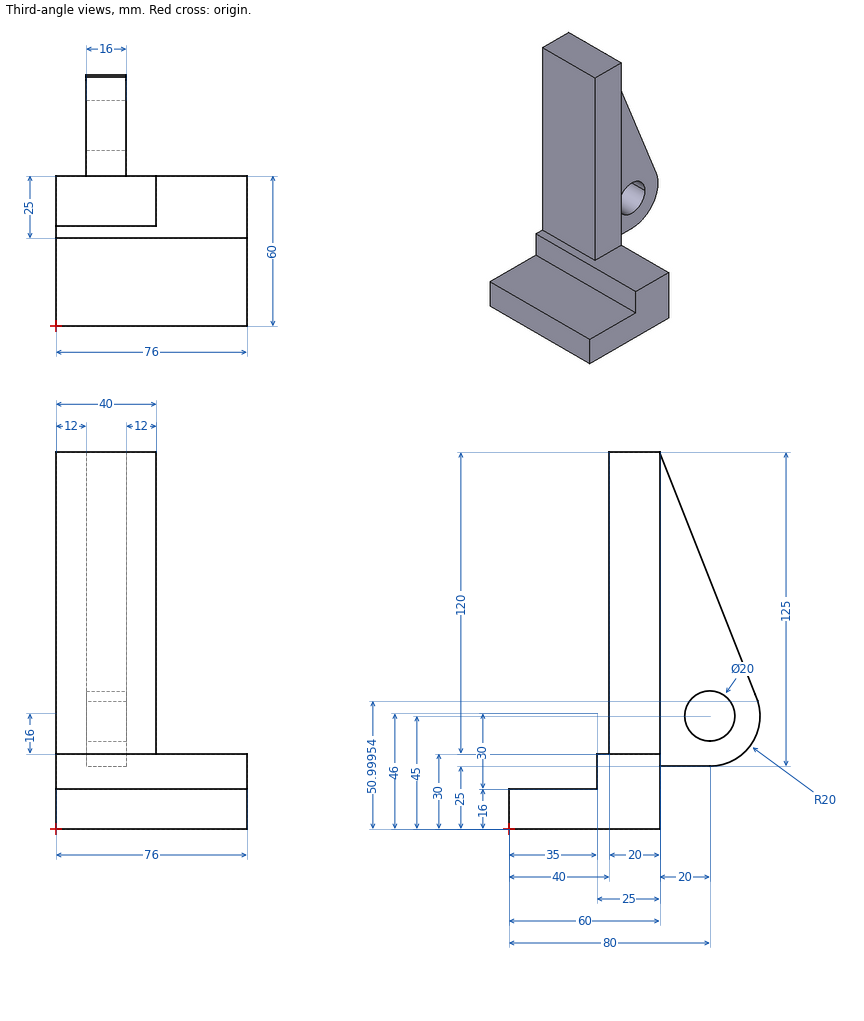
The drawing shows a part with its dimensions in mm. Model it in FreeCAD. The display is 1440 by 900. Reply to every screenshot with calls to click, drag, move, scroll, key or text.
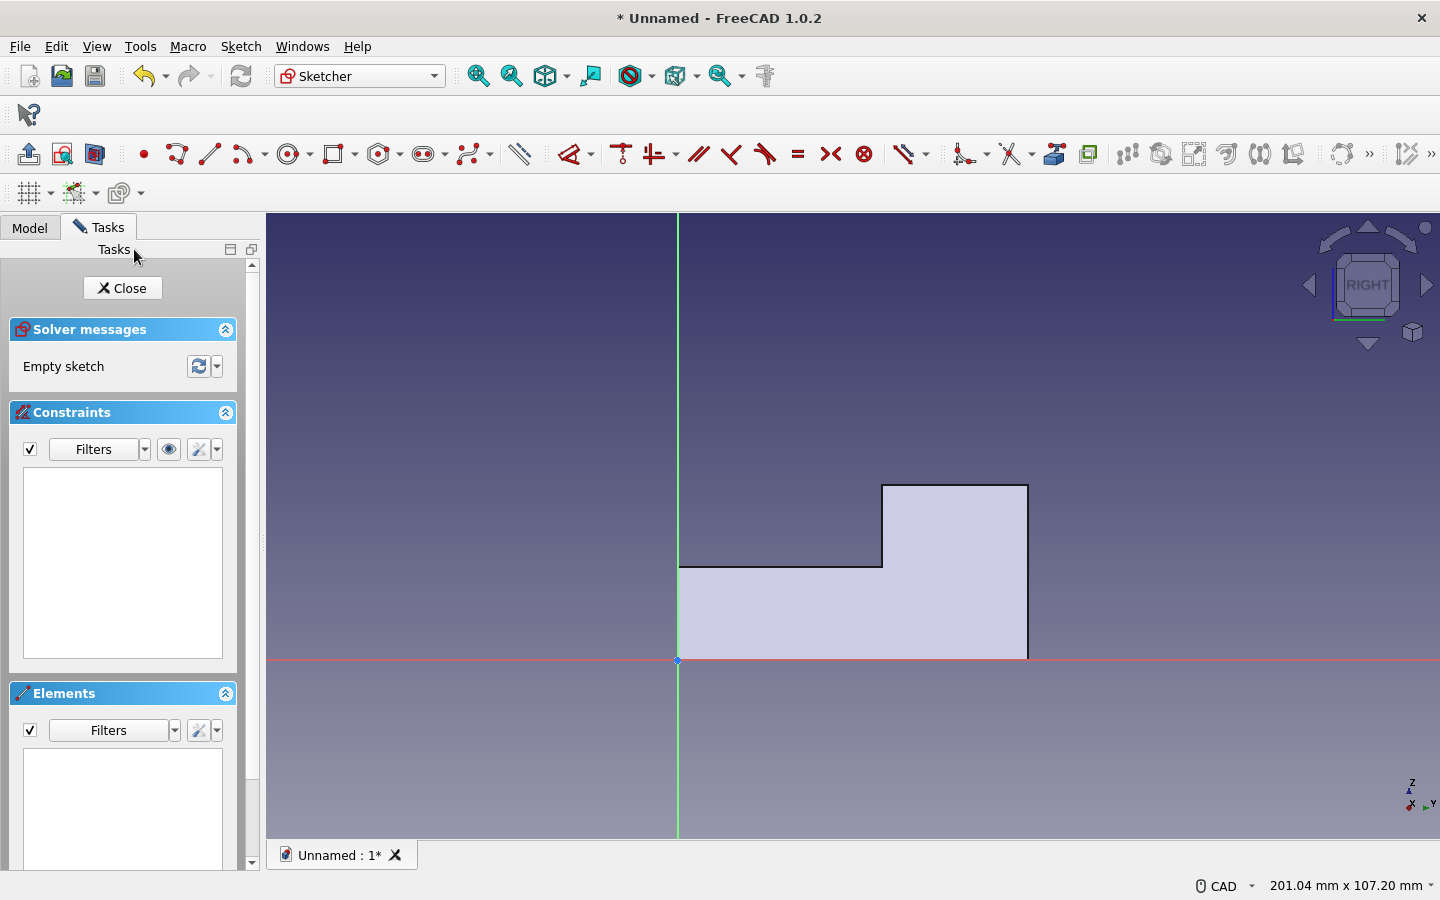
scroll(729, 774, down, 4)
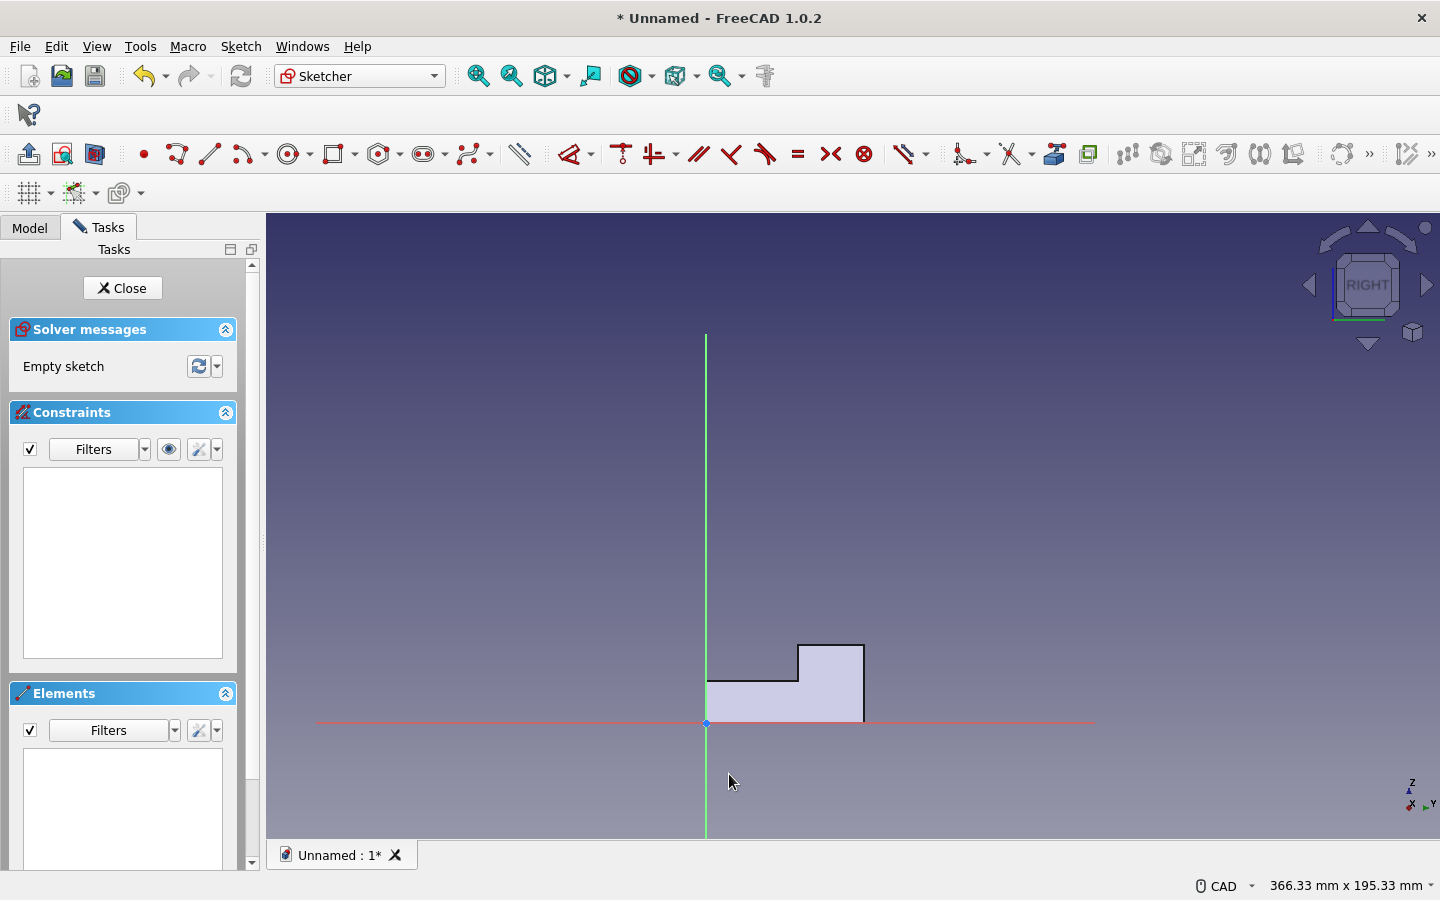
key(g)
key(r)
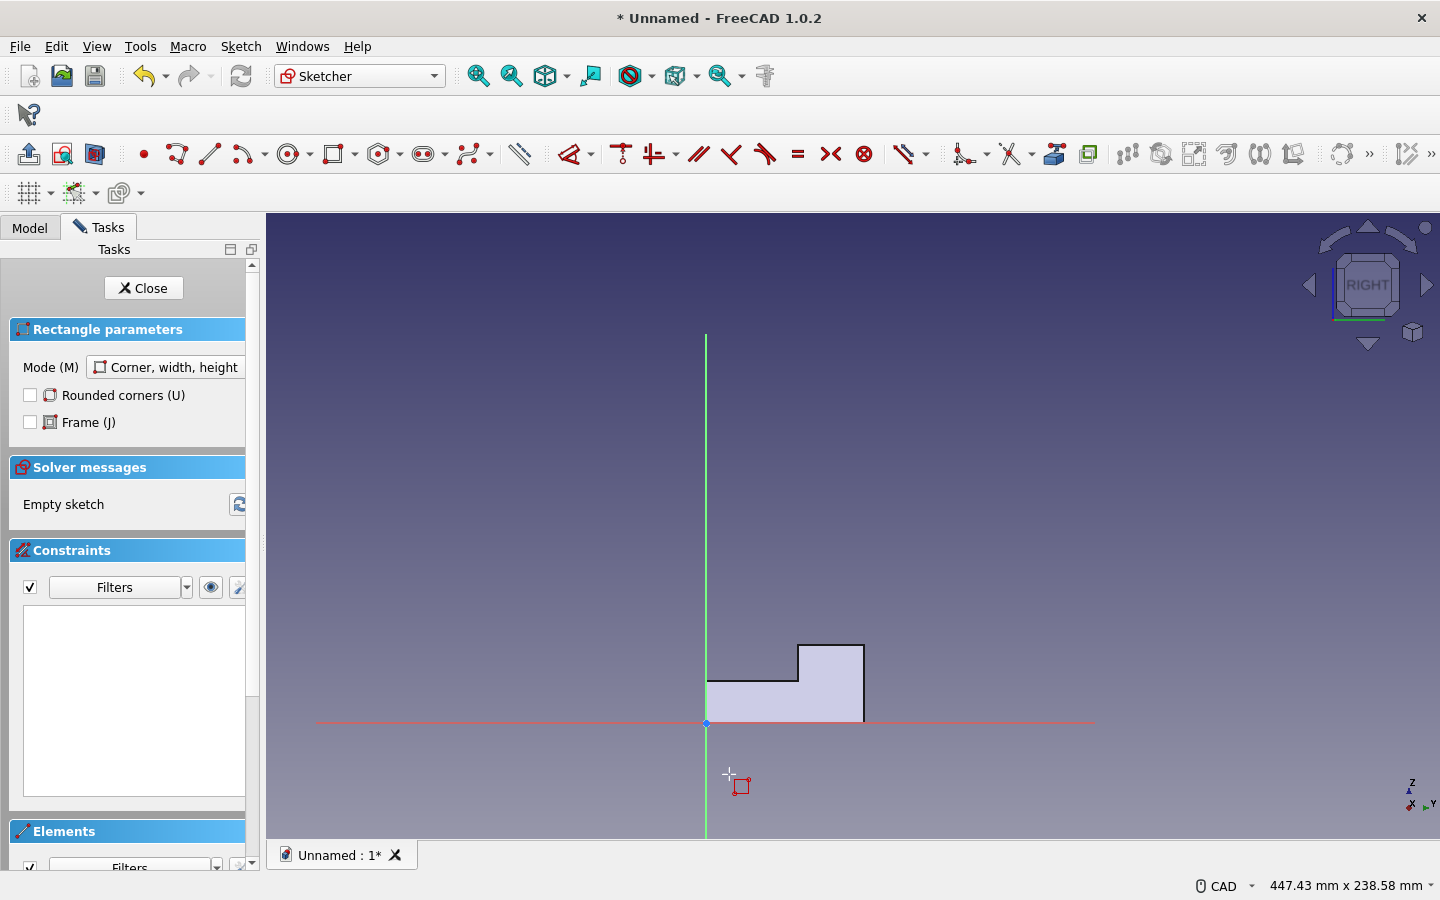
click(811, 330)
click(864, 645)
key(Escape)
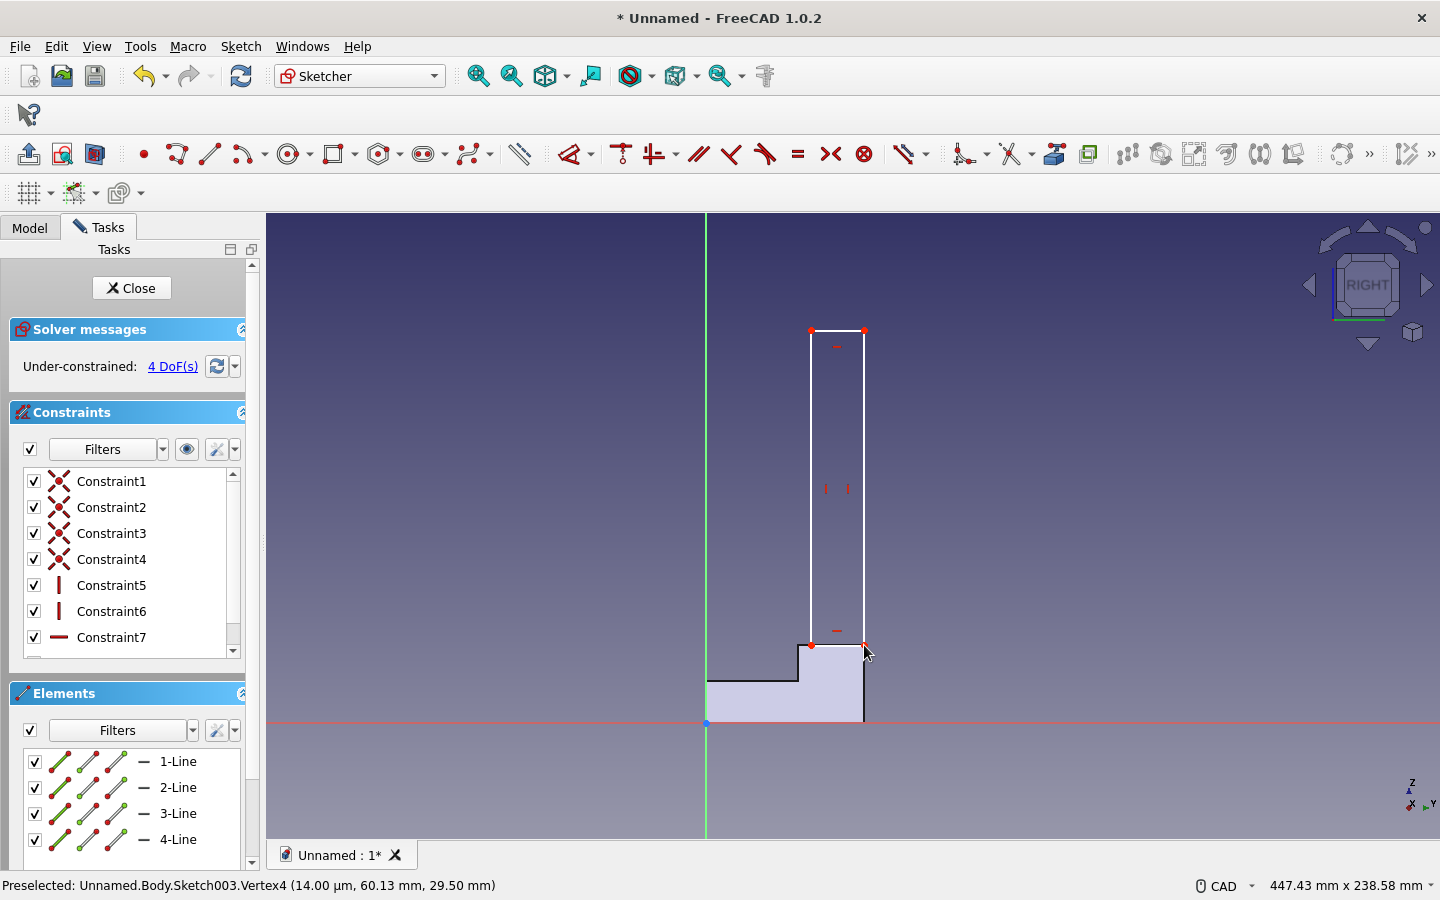
click(568, 154)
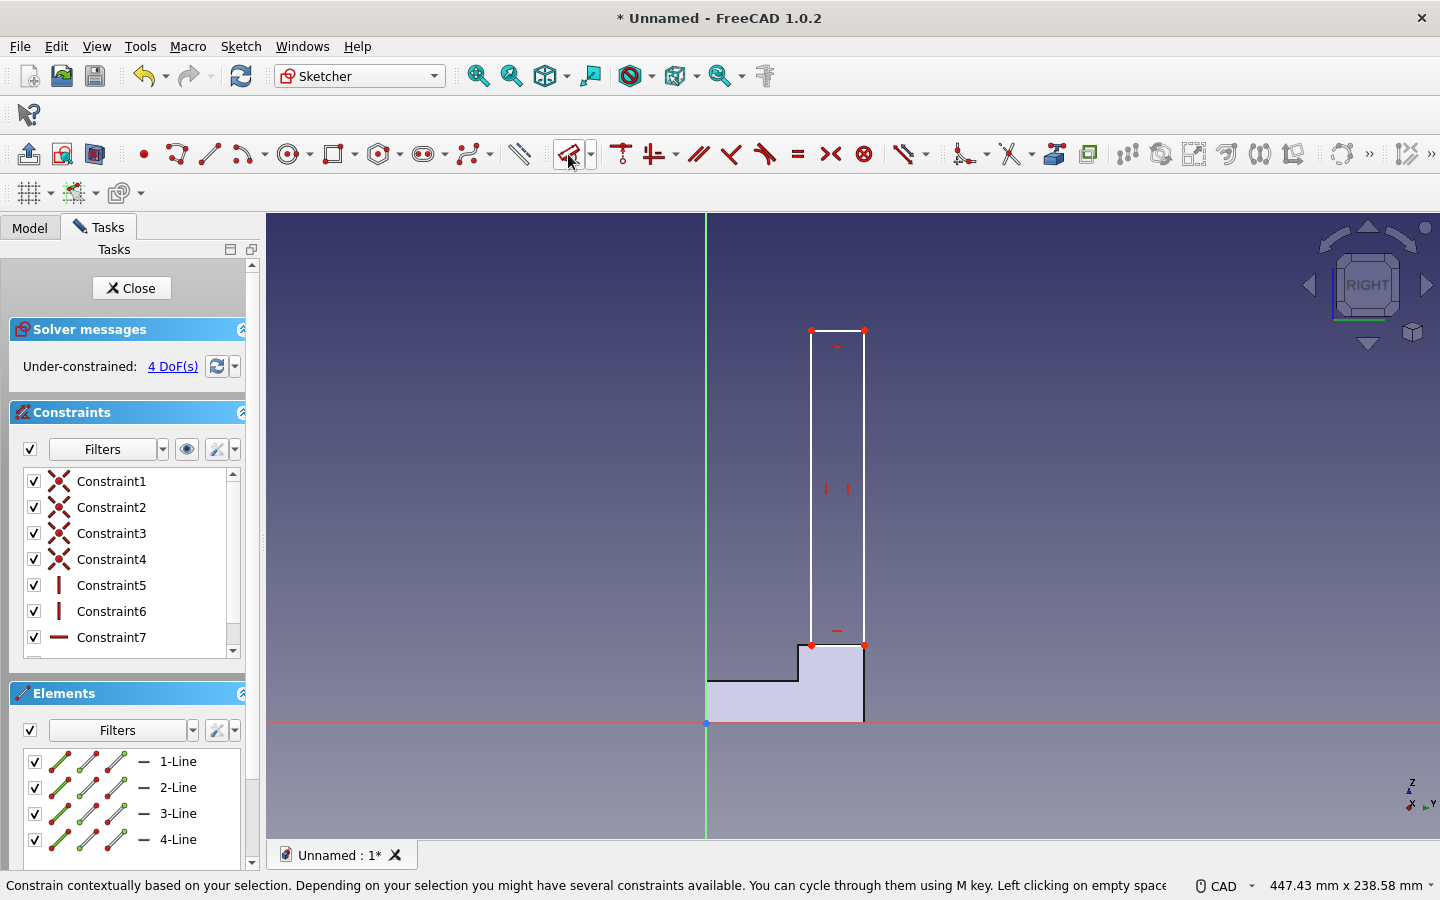
click(827, 646)
click(837, 680)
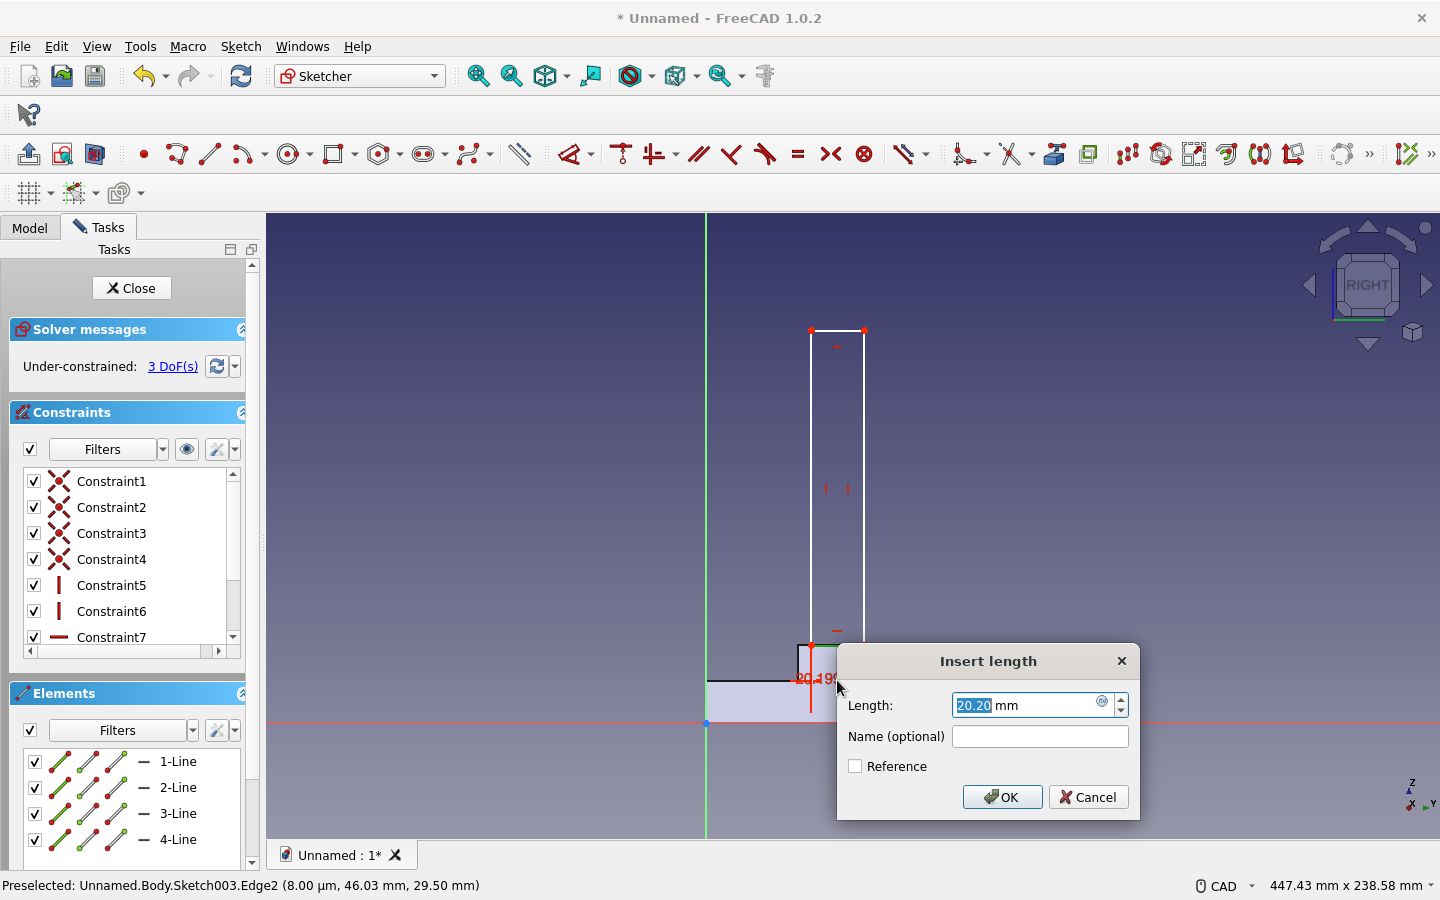
text(20)
key(Return)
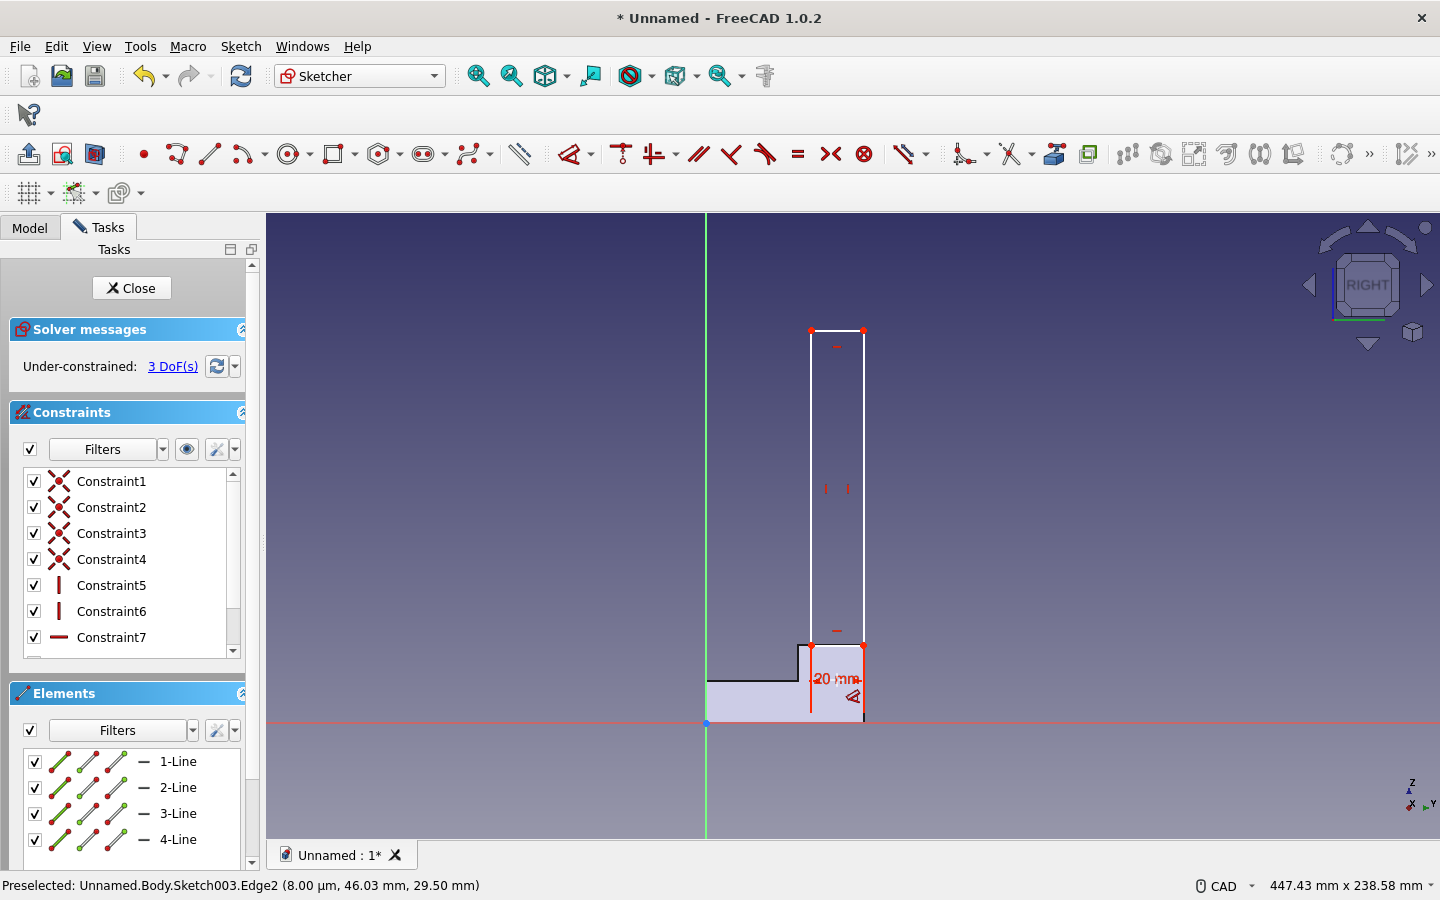
click(811, 425)
click(845, 488)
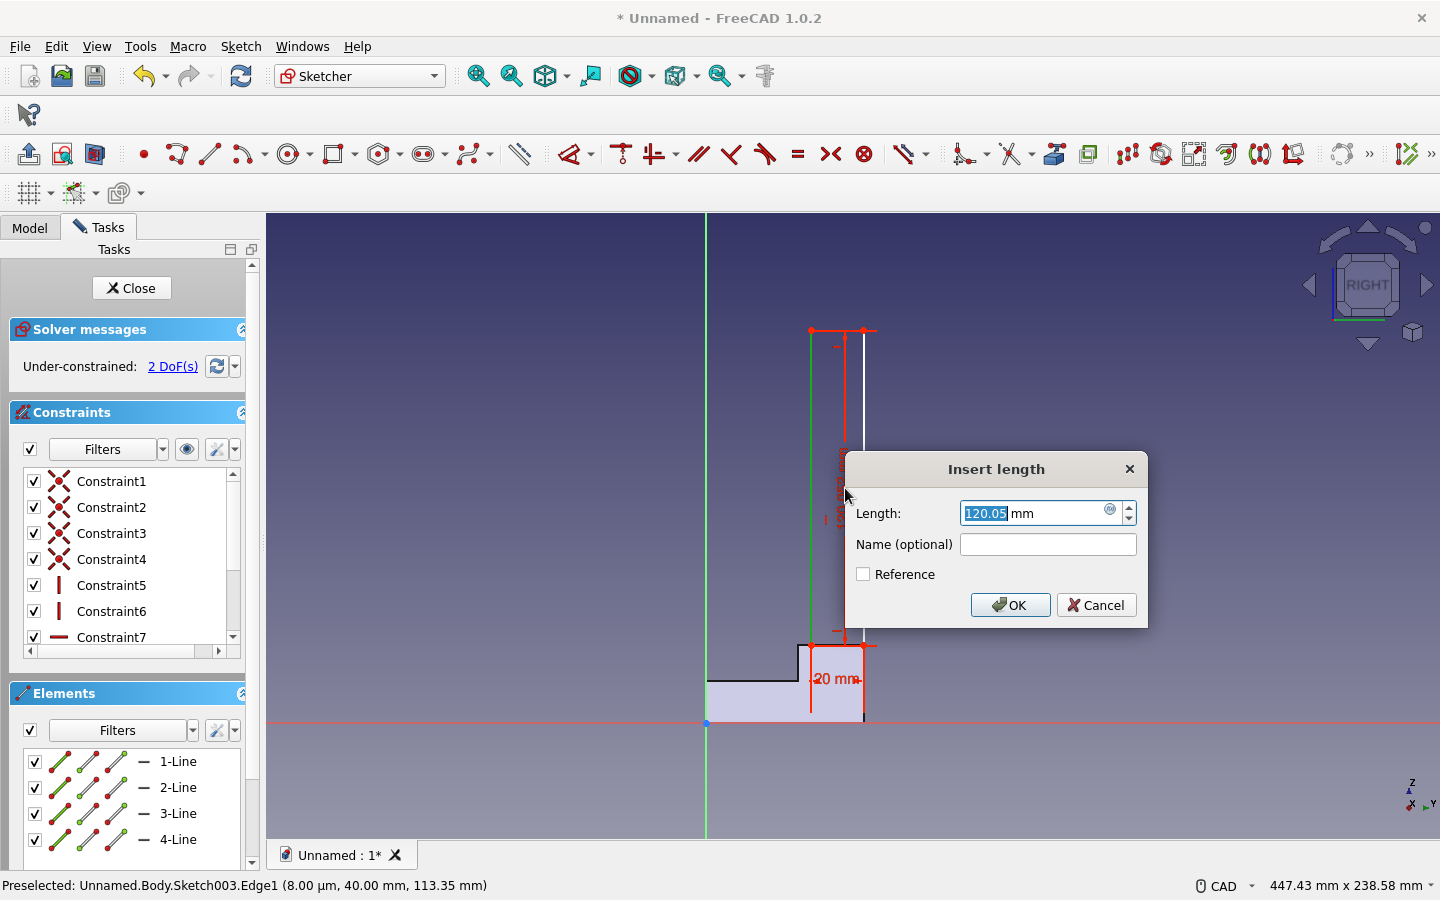
text(120)
key(Return)